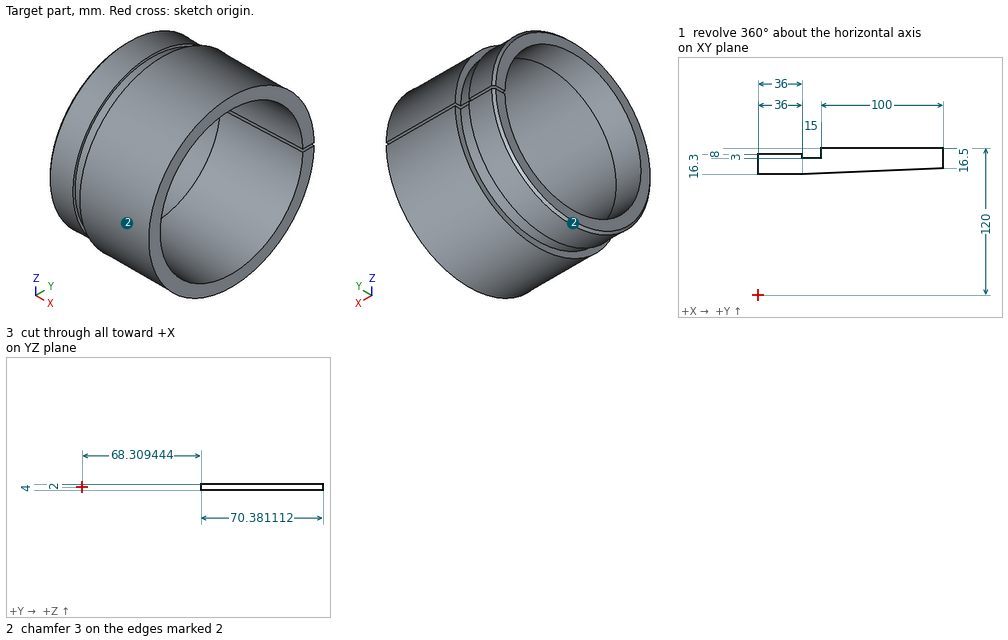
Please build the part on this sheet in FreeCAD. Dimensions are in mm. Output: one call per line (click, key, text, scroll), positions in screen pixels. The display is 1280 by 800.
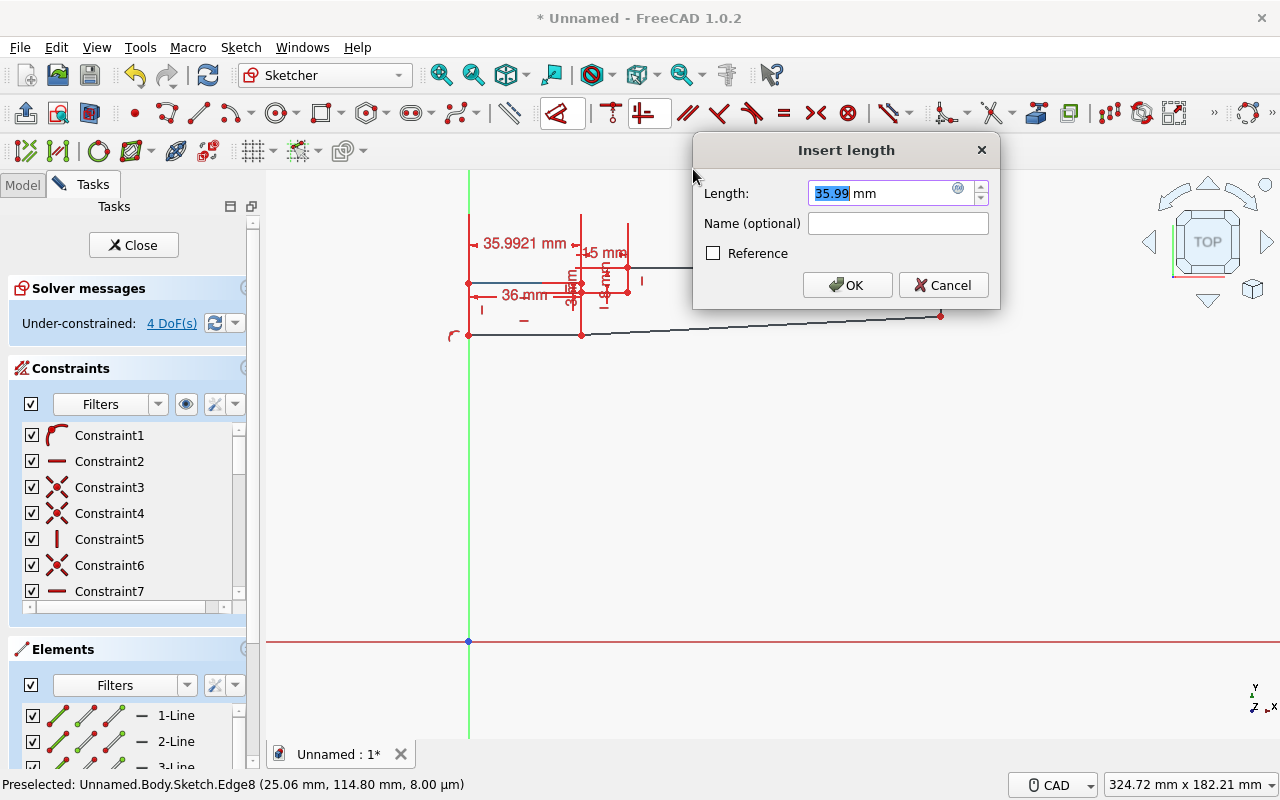
text(36)
key(Return)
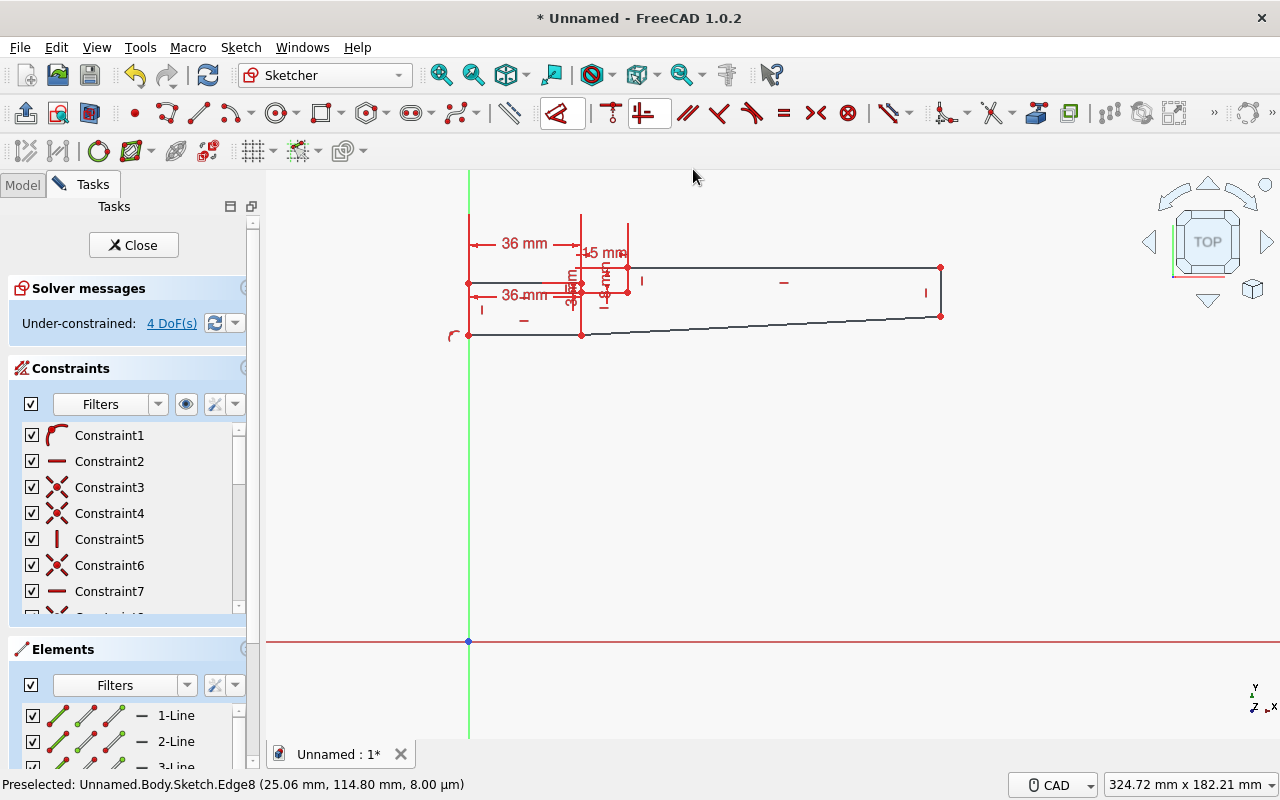
click(847, 268)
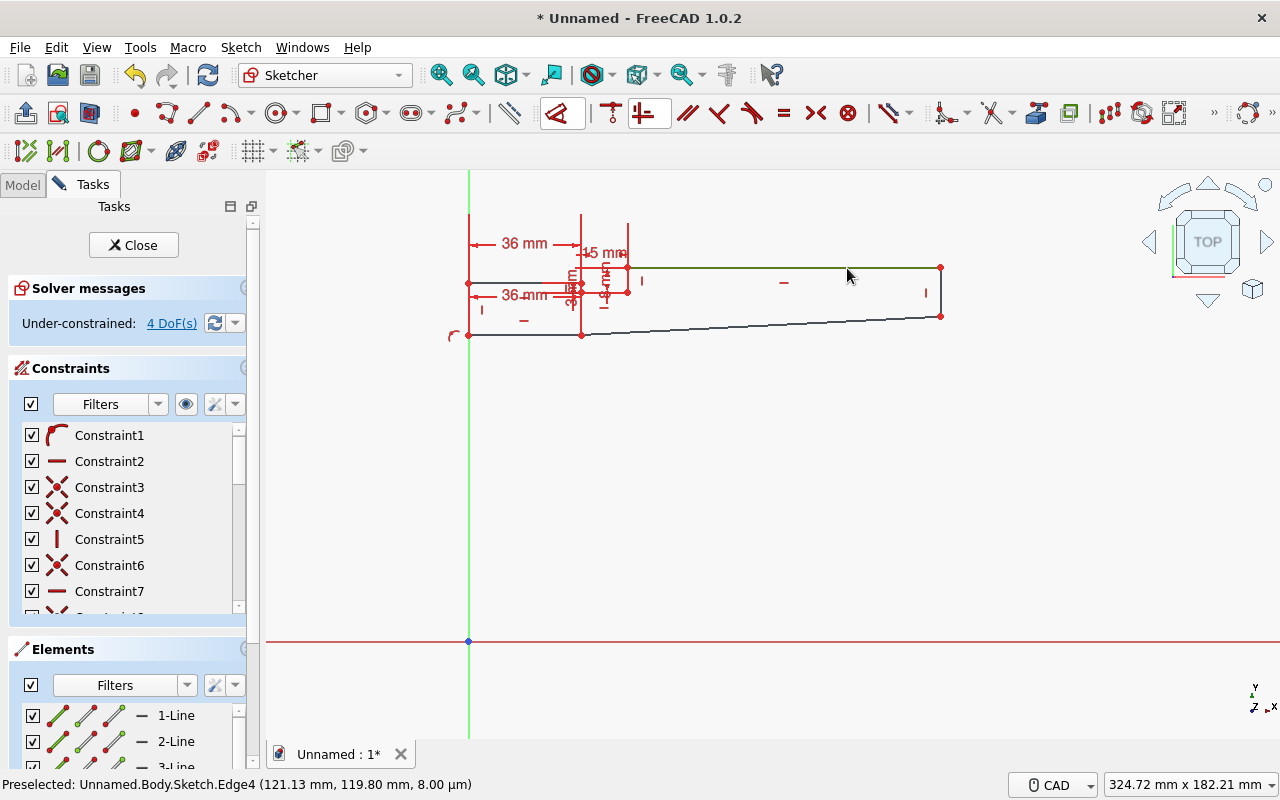
click(580, 114)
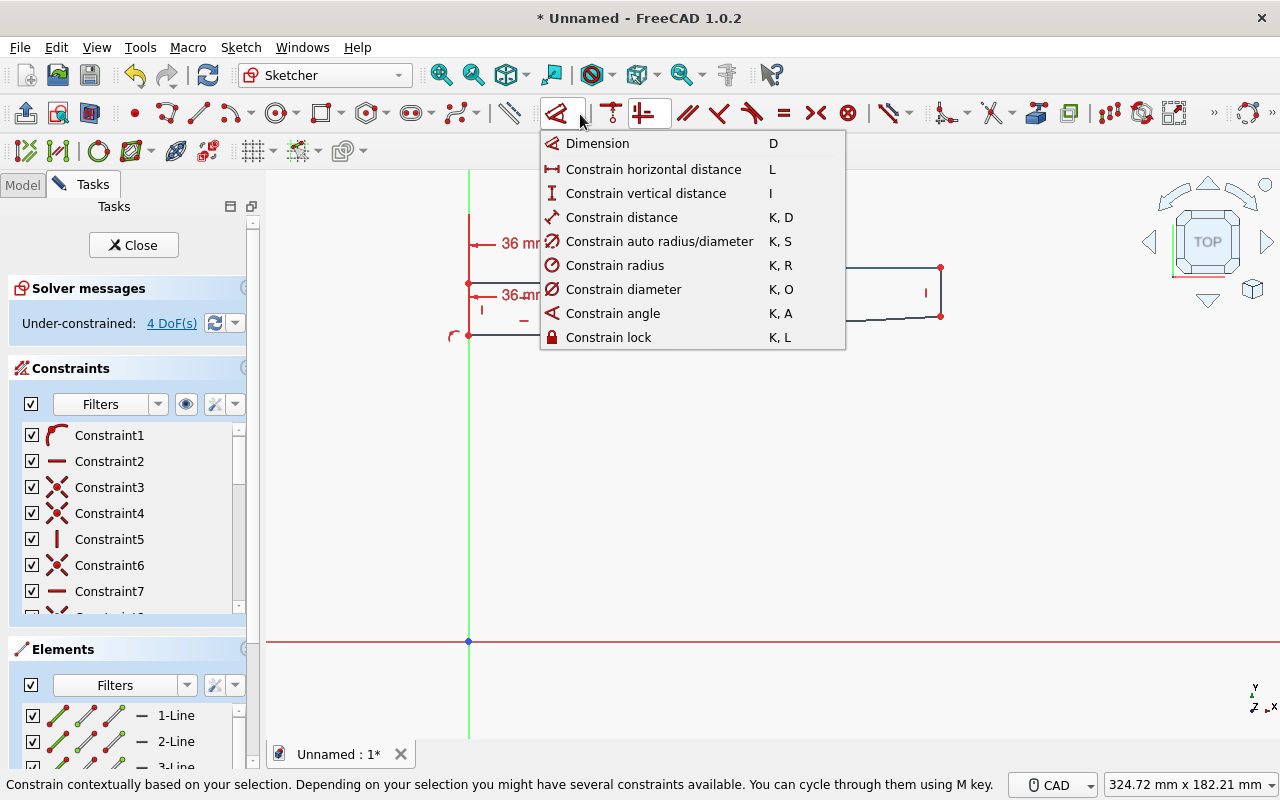
click(693, 169)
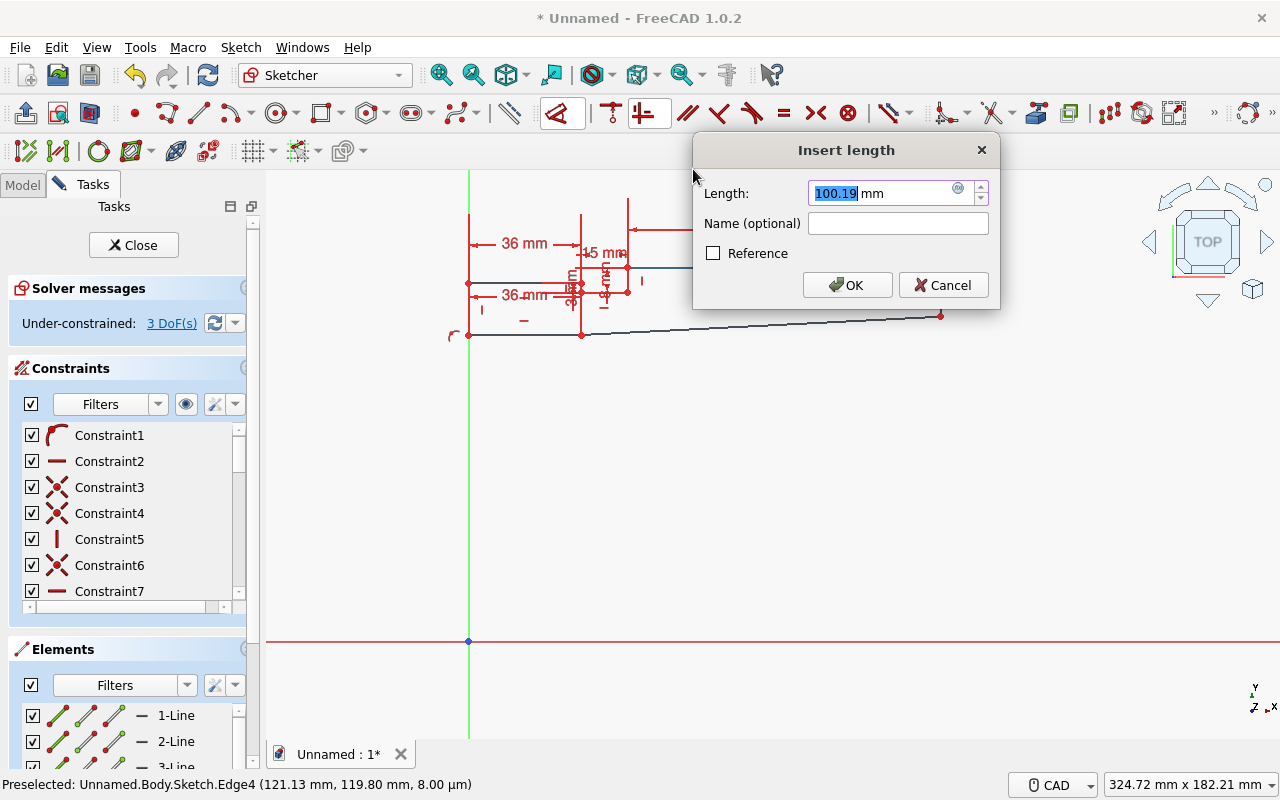
text(100)
key(Return)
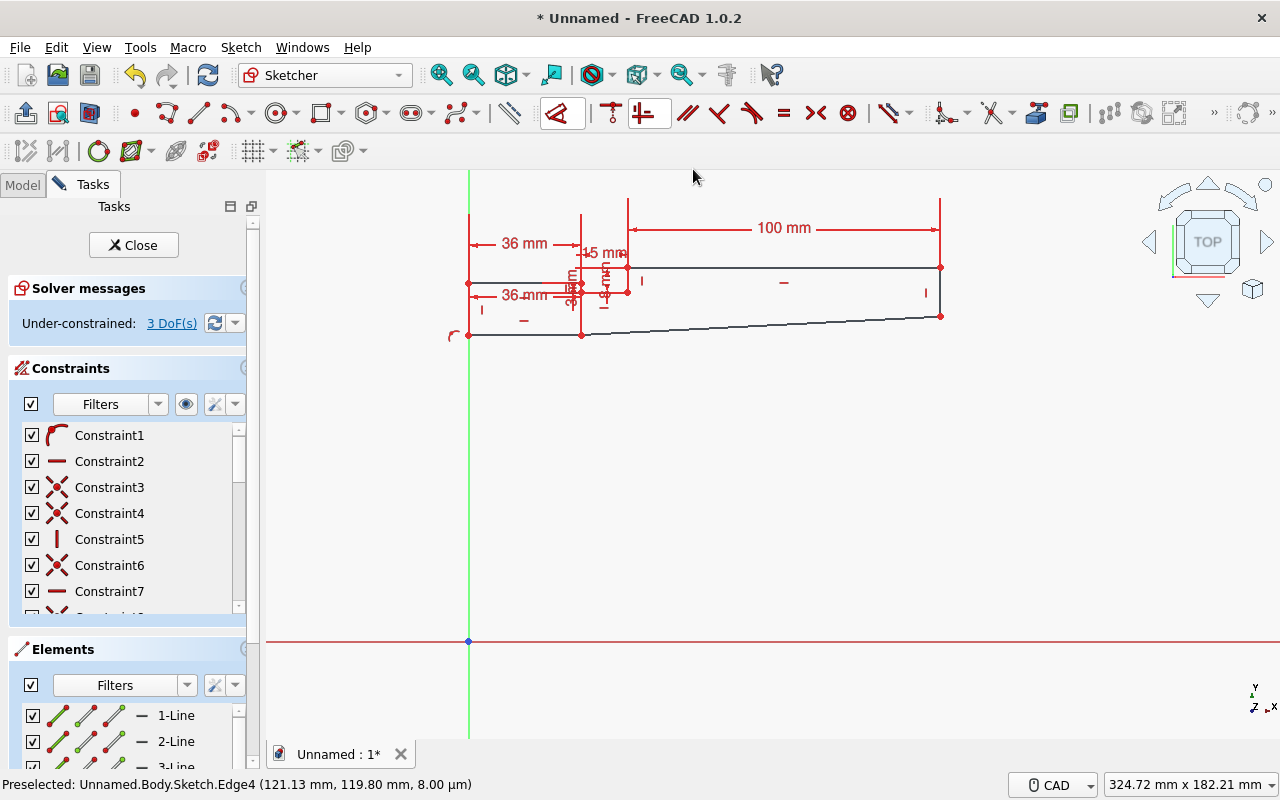
click(940, 302)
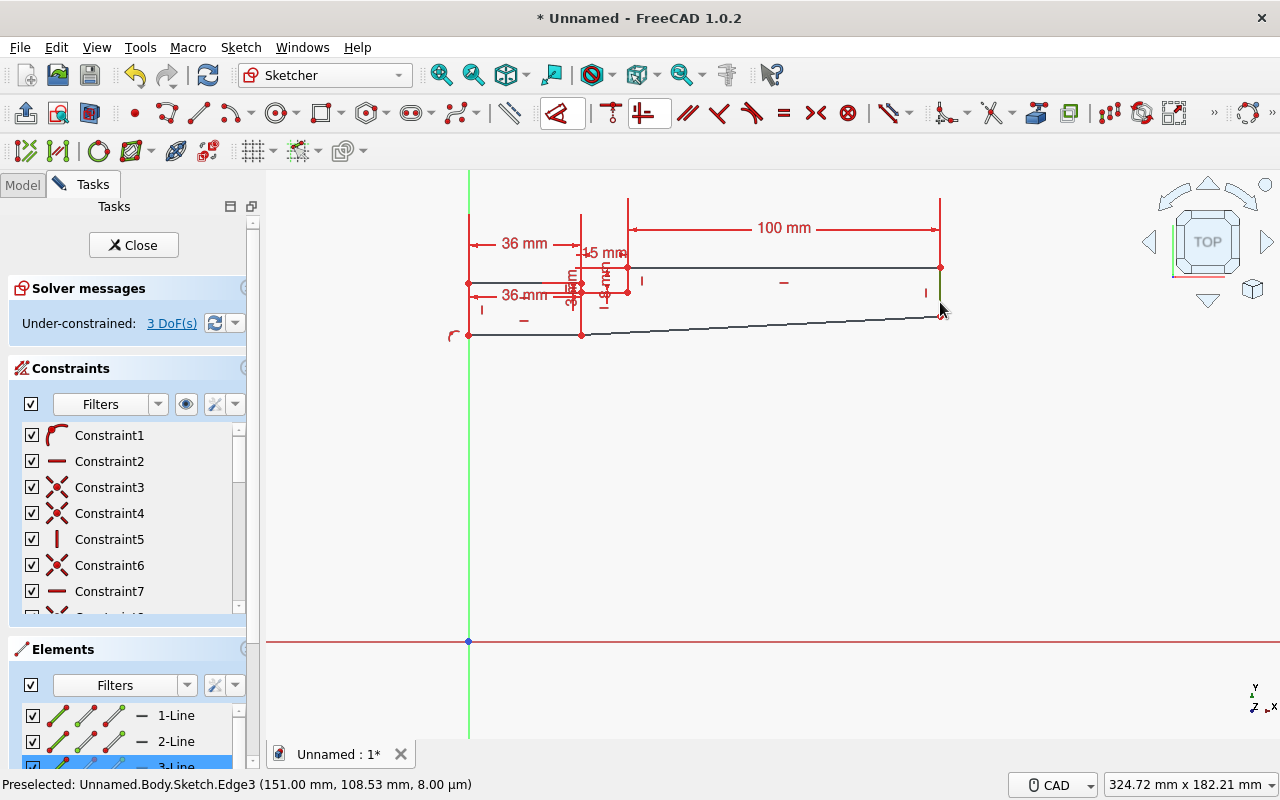
key(i)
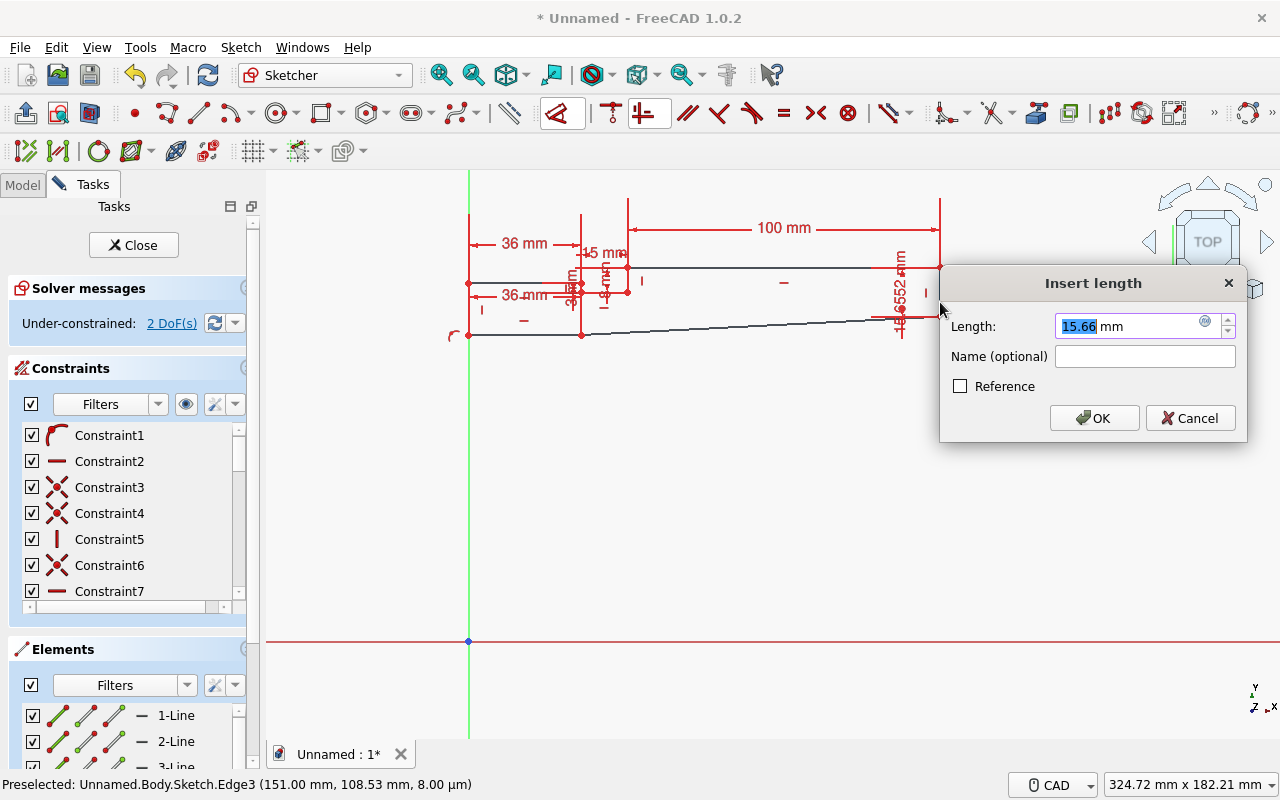
text(16.5)
key(Return)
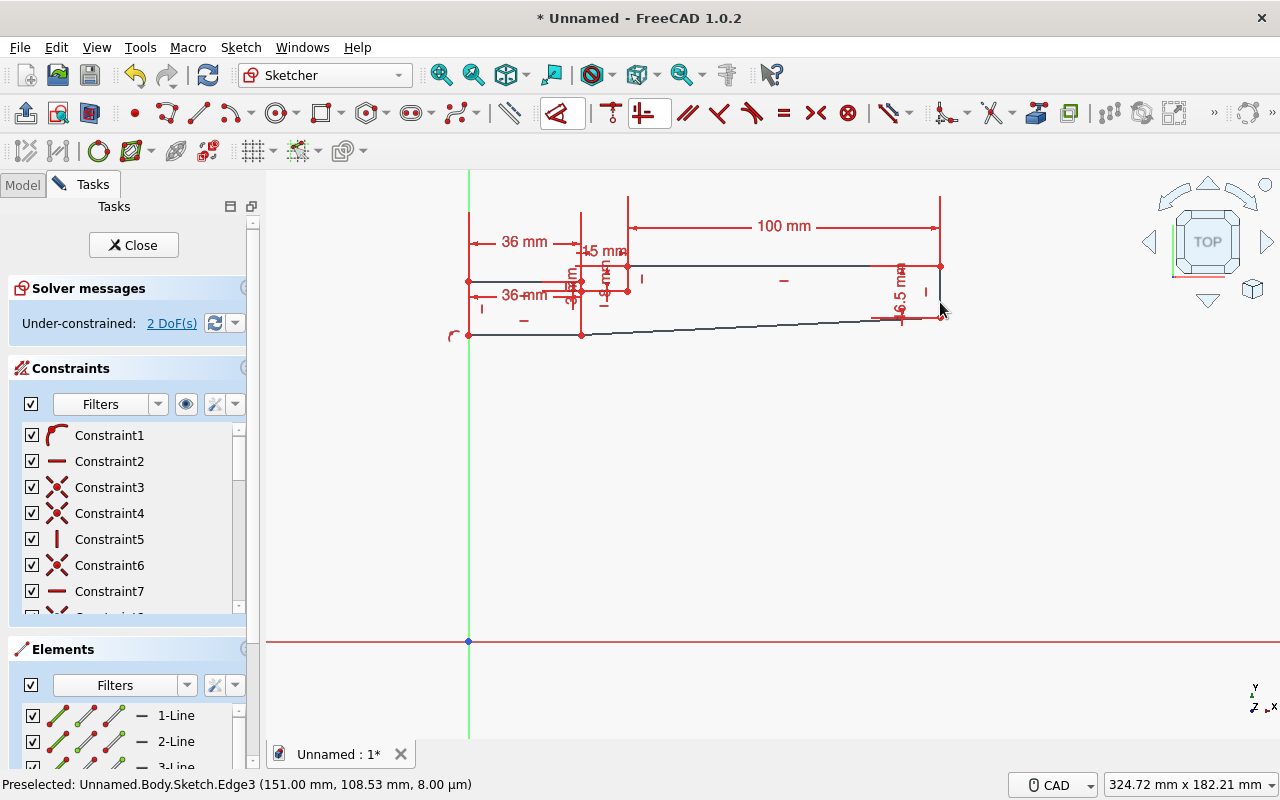
click(469, 298)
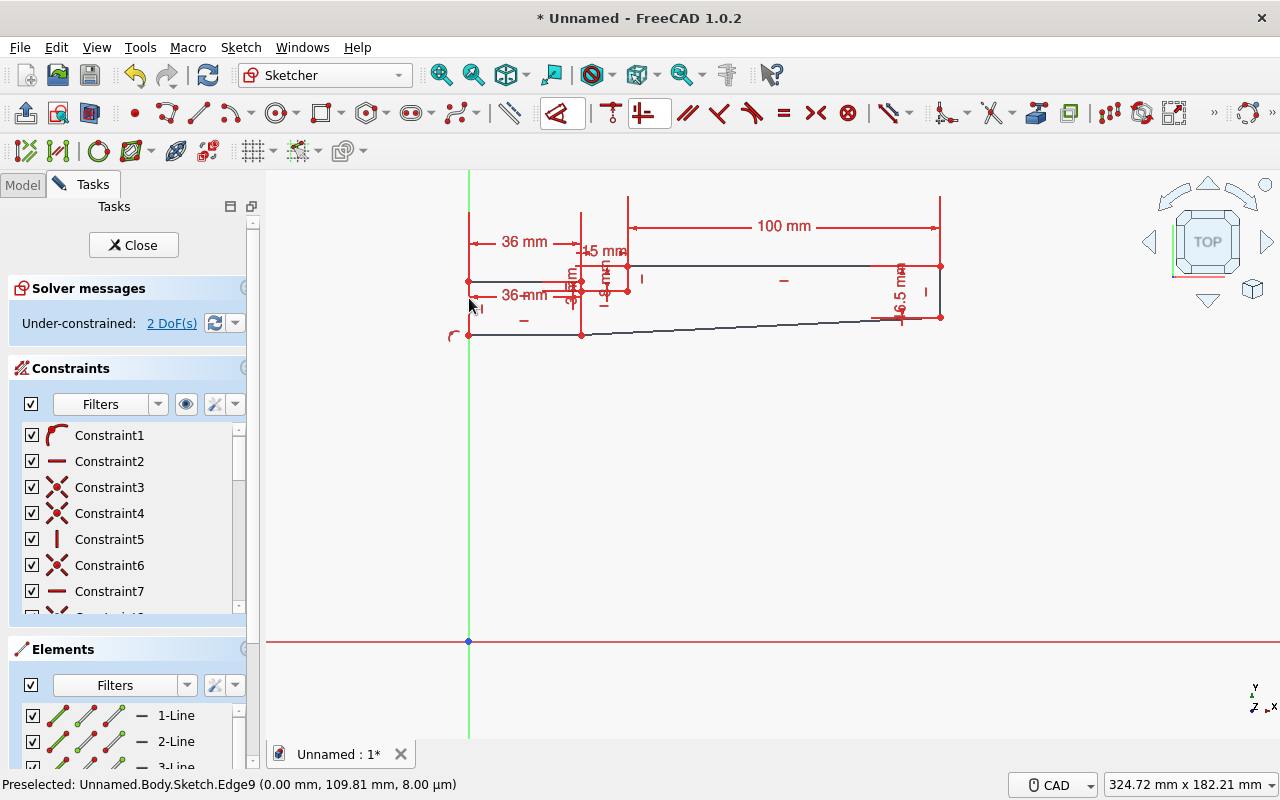
click(580, 114)